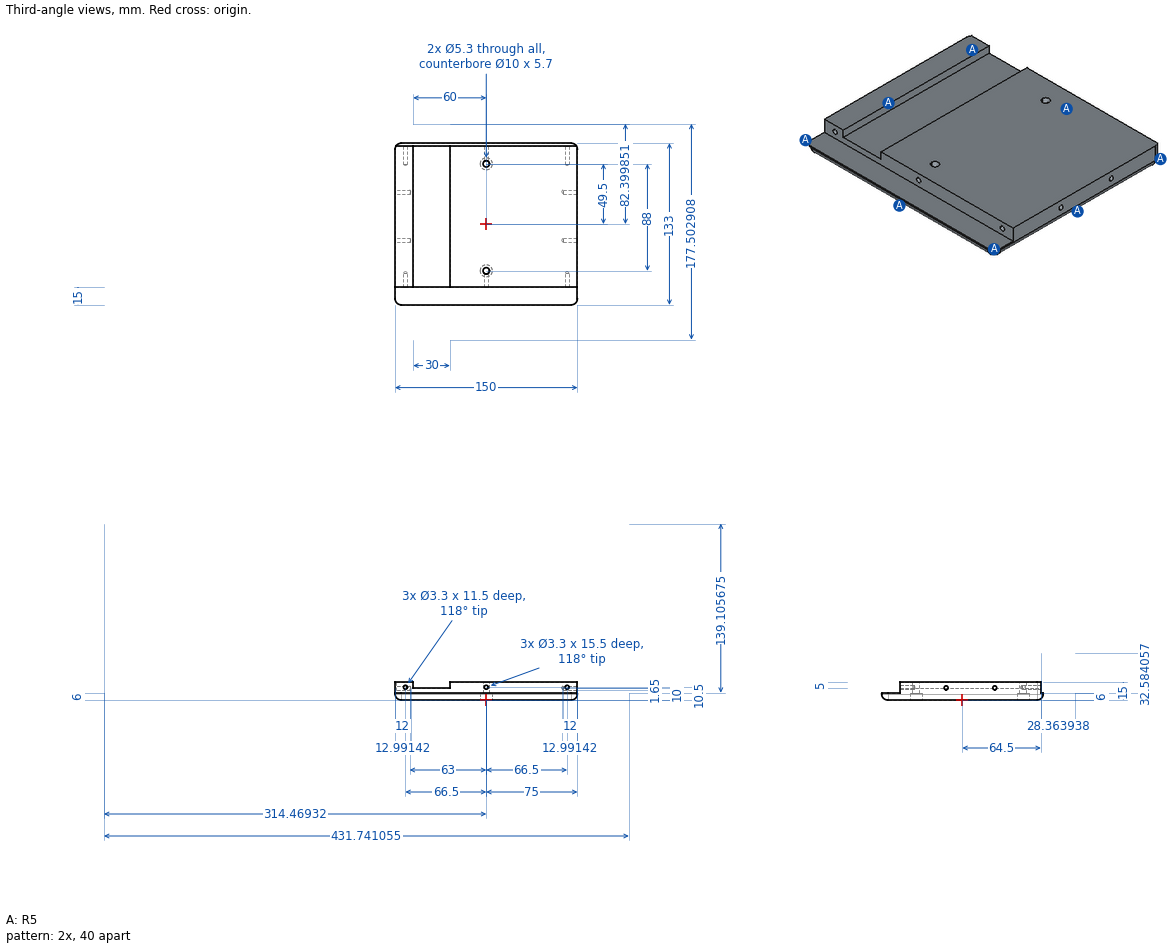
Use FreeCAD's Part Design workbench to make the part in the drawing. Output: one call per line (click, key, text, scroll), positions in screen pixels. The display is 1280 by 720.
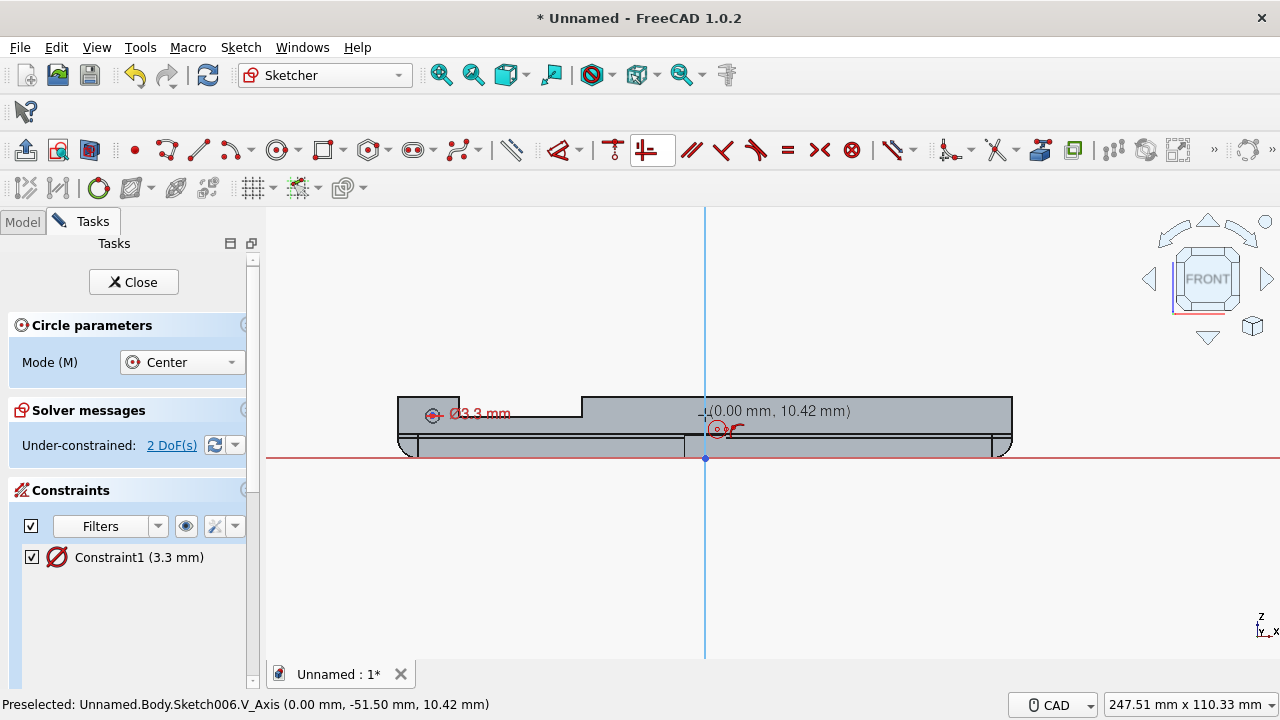
click(705, 415)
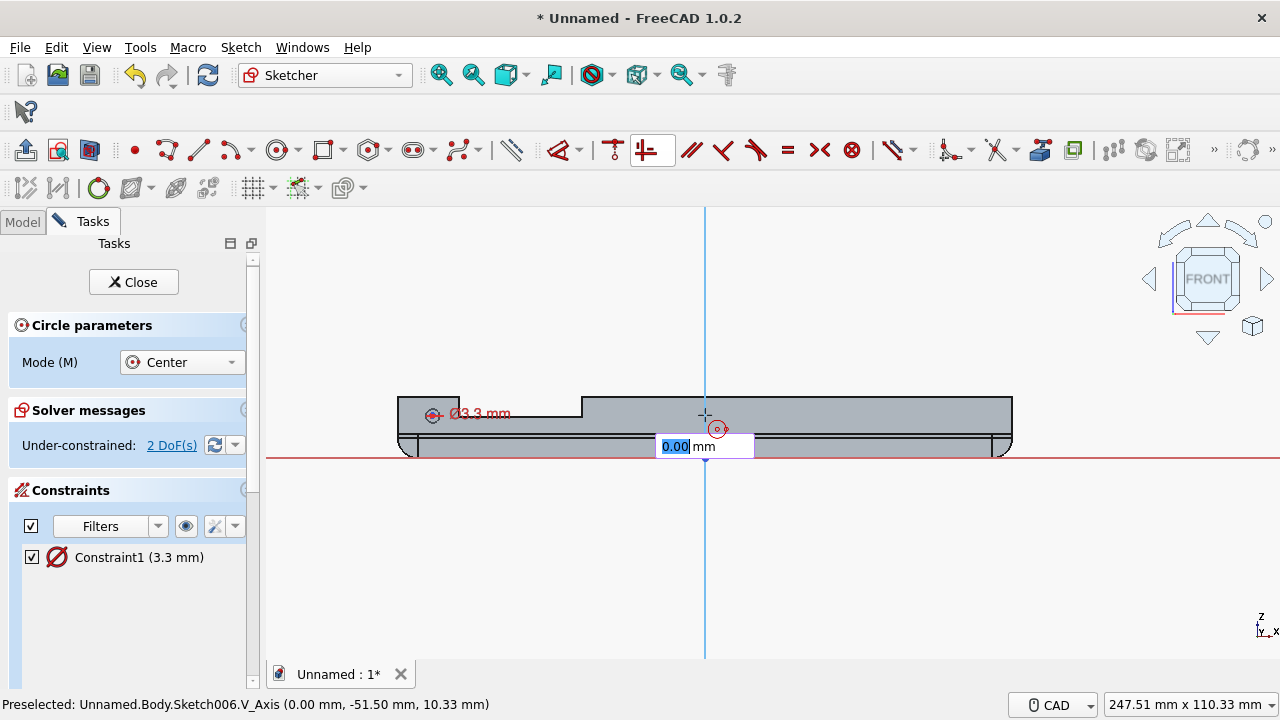
scroll(711, 413, up, 5)
move(711, 412)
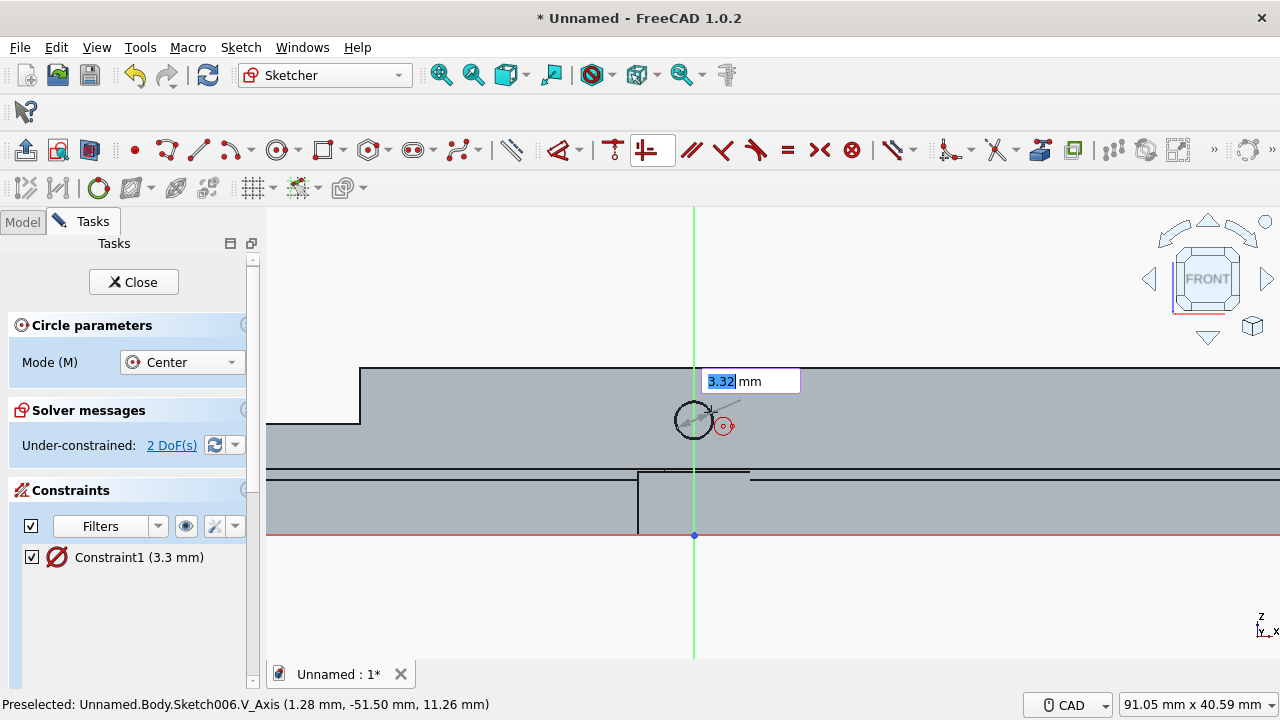
text(3.3)
key(Return)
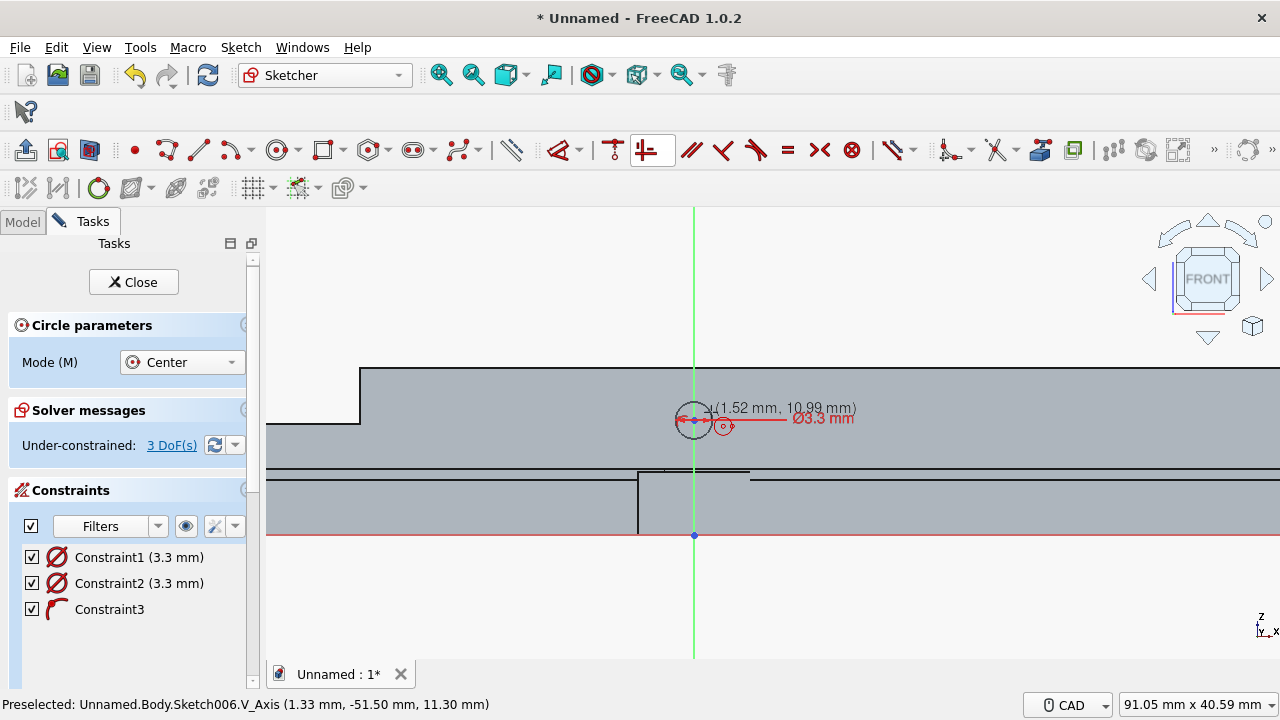
scroll(711, 413, down, 5)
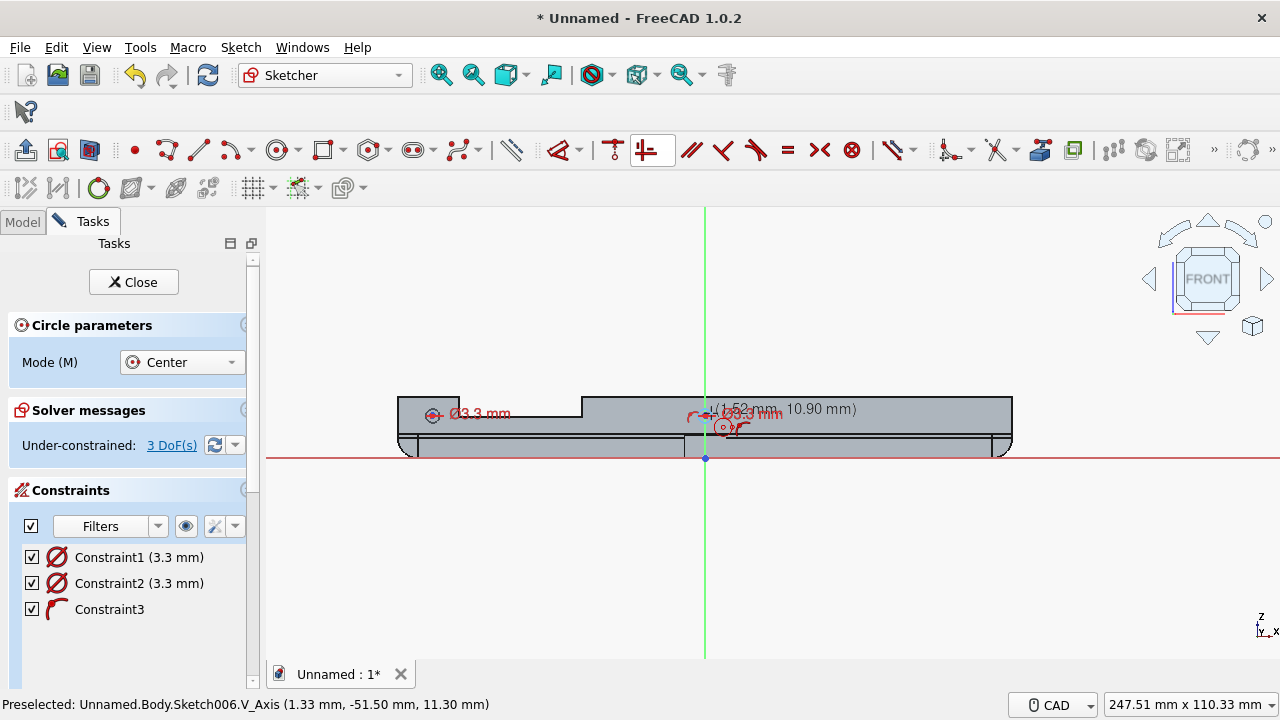
scroll(977, 415, up, 7)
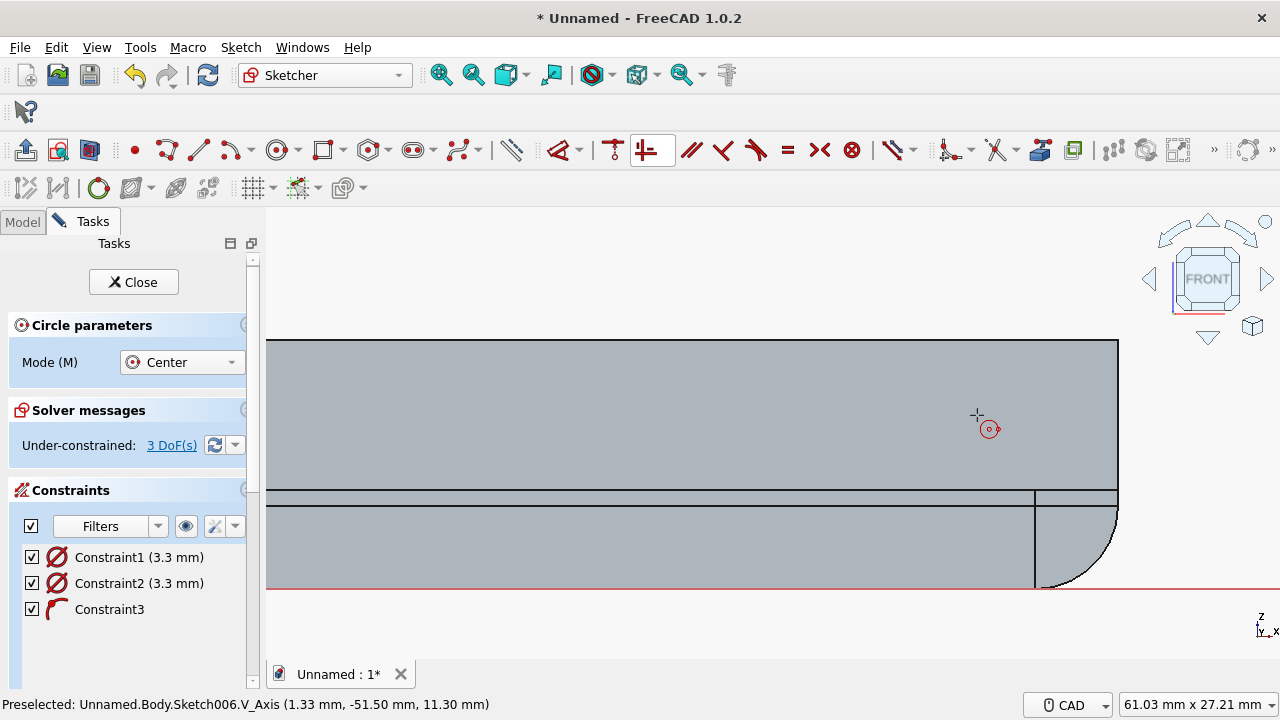
scroll(977, 415, down, 7)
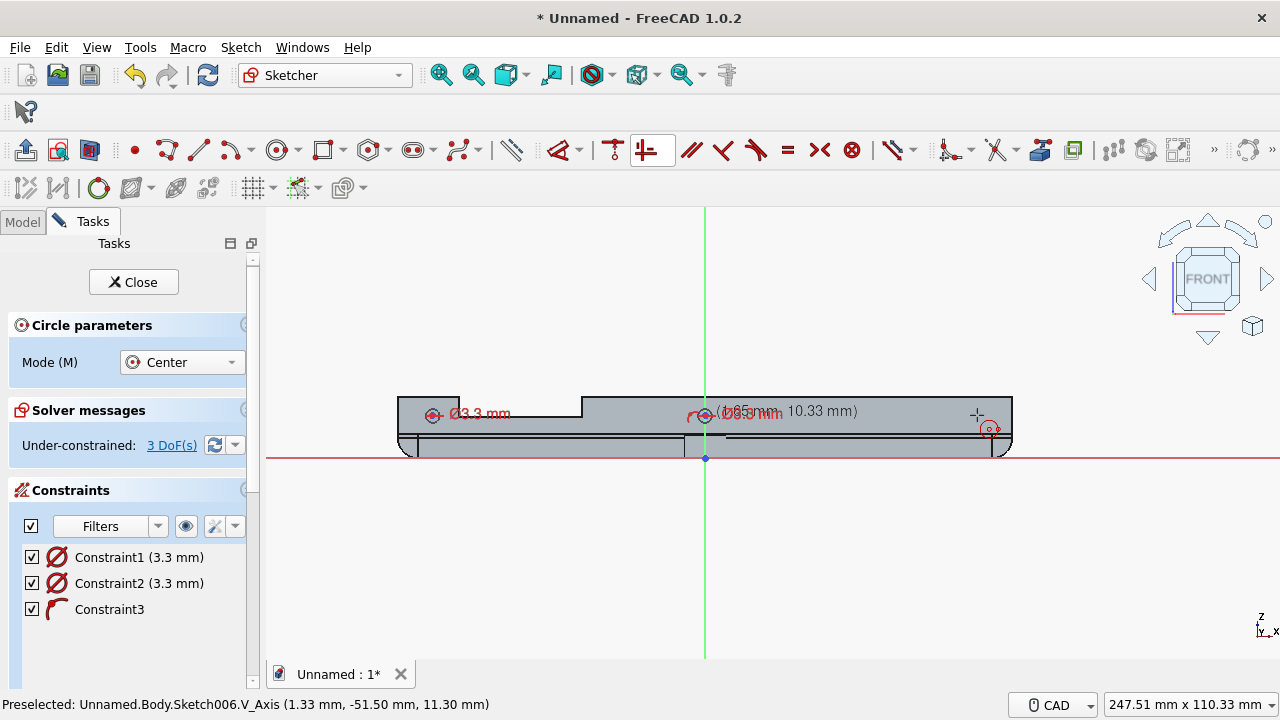
click(977, 415)
move(982, 411)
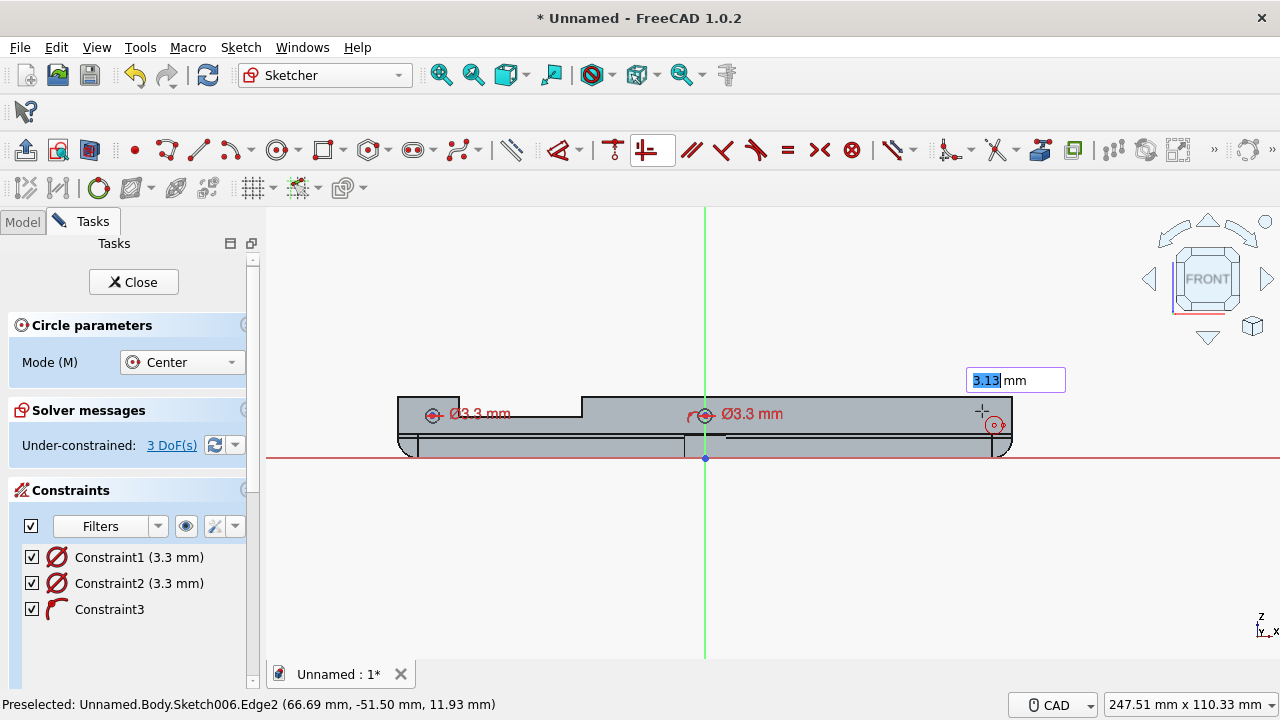
text(3.3)
key(Return)
key(Escape)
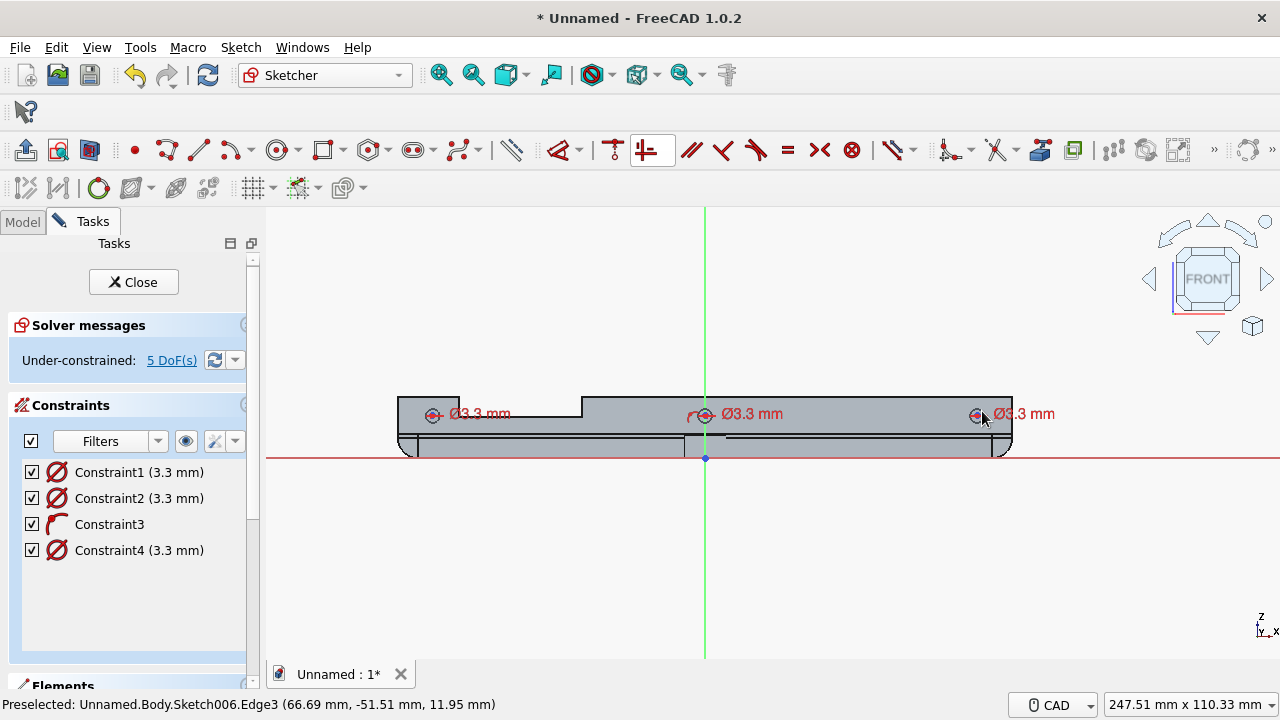
click(433, 416)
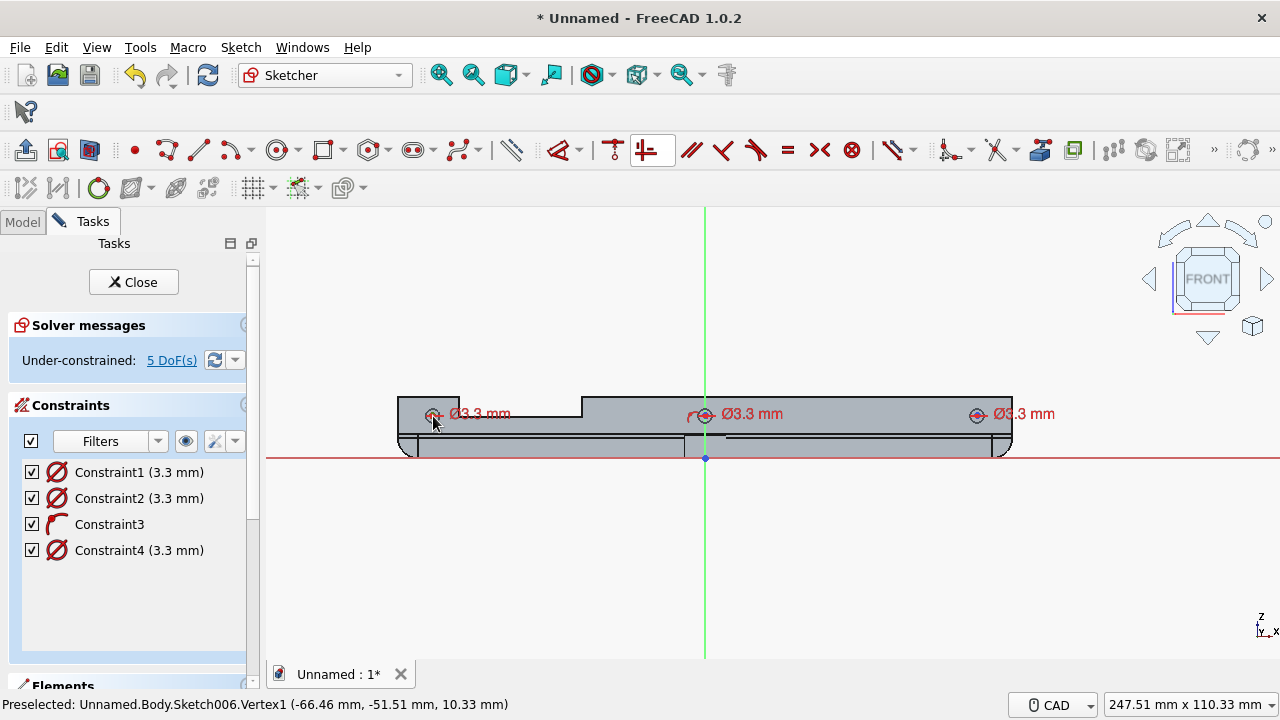
click(705, 416)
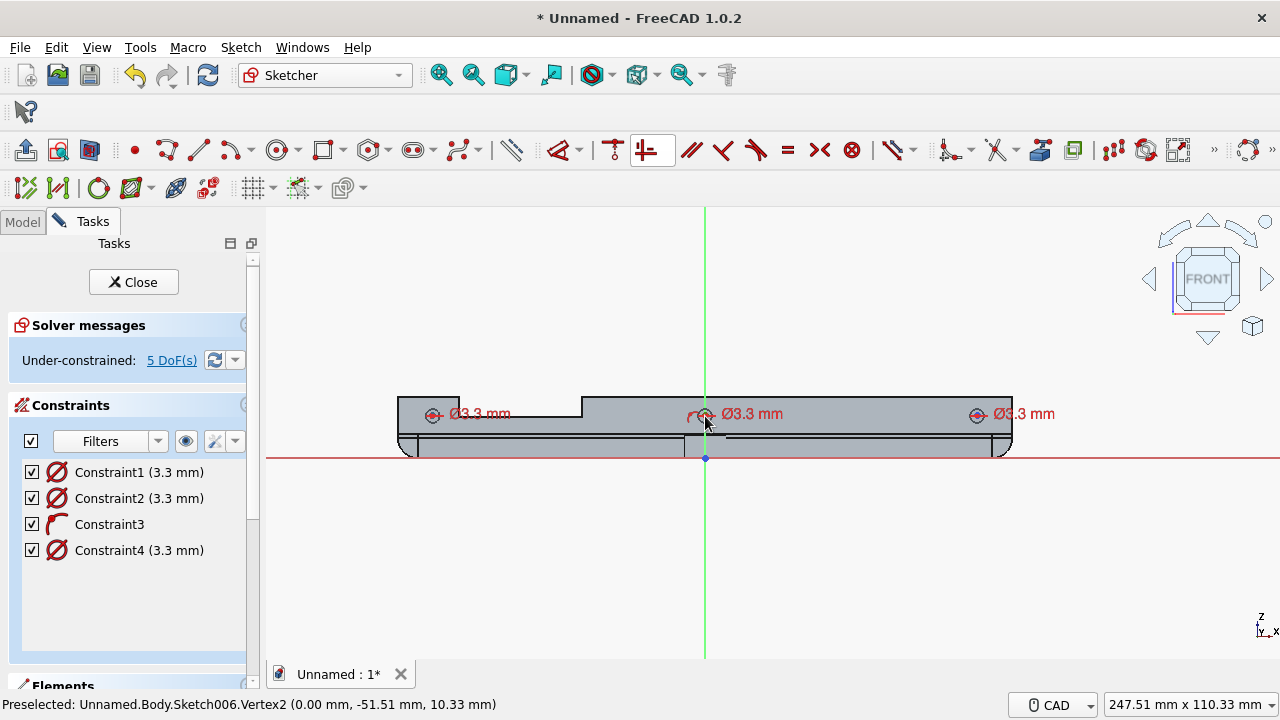
click(670, 150)